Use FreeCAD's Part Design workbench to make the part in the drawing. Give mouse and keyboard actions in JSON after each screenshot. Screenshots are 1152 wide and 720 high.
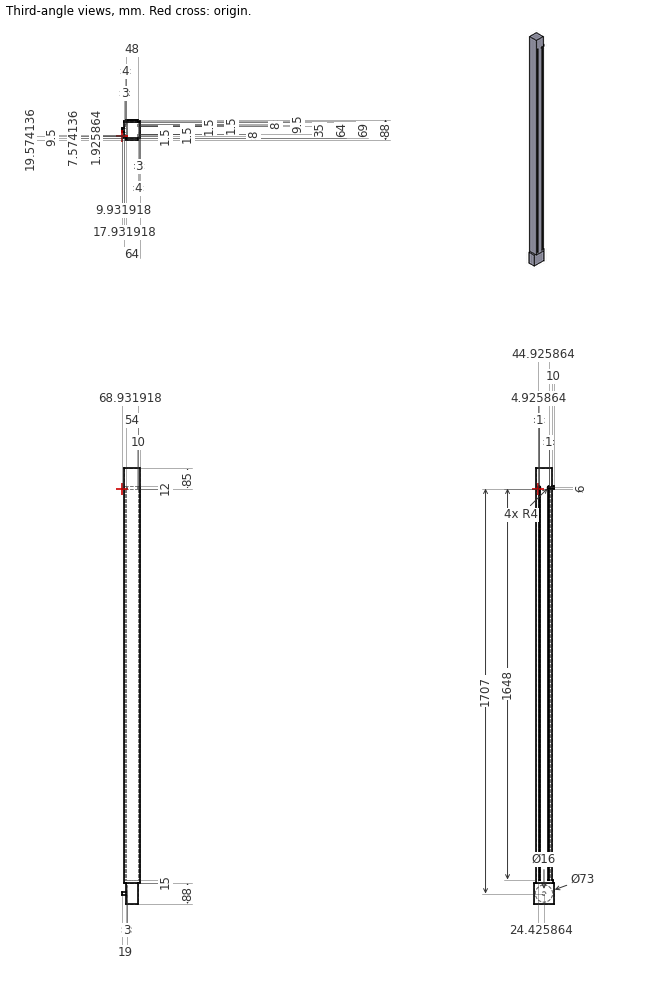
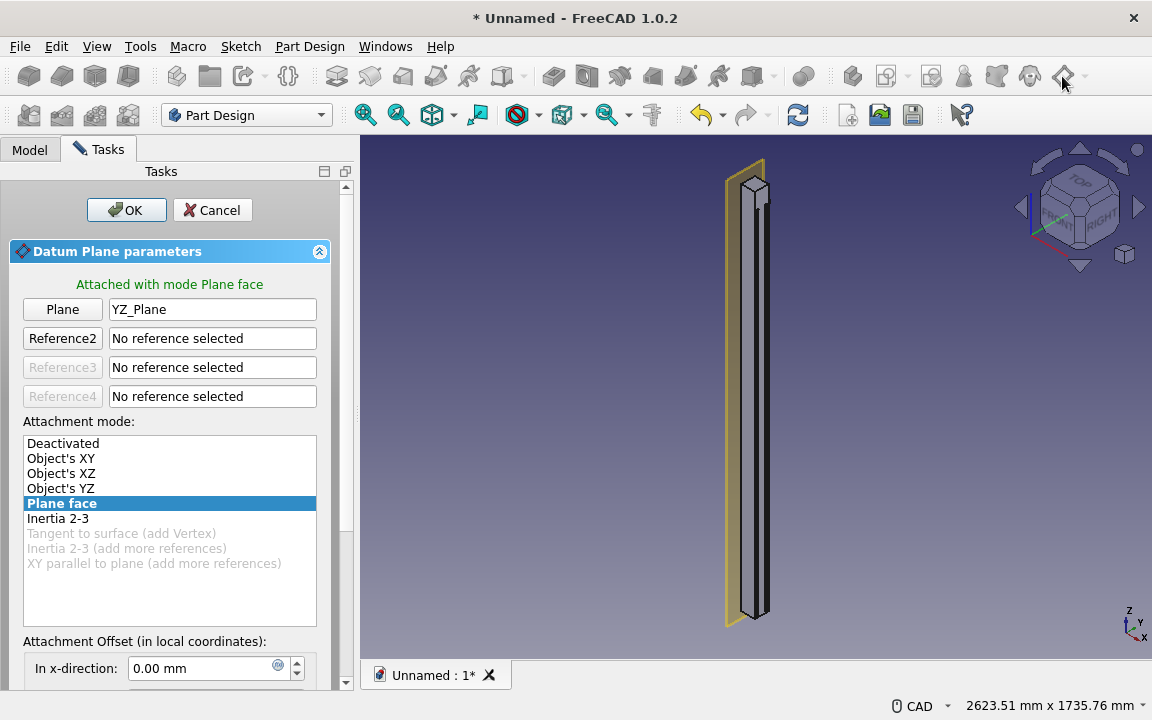
{"action": "scroll", "coordinate": [346, 436], "scroll_direction": "down", "scroll_amount": 2}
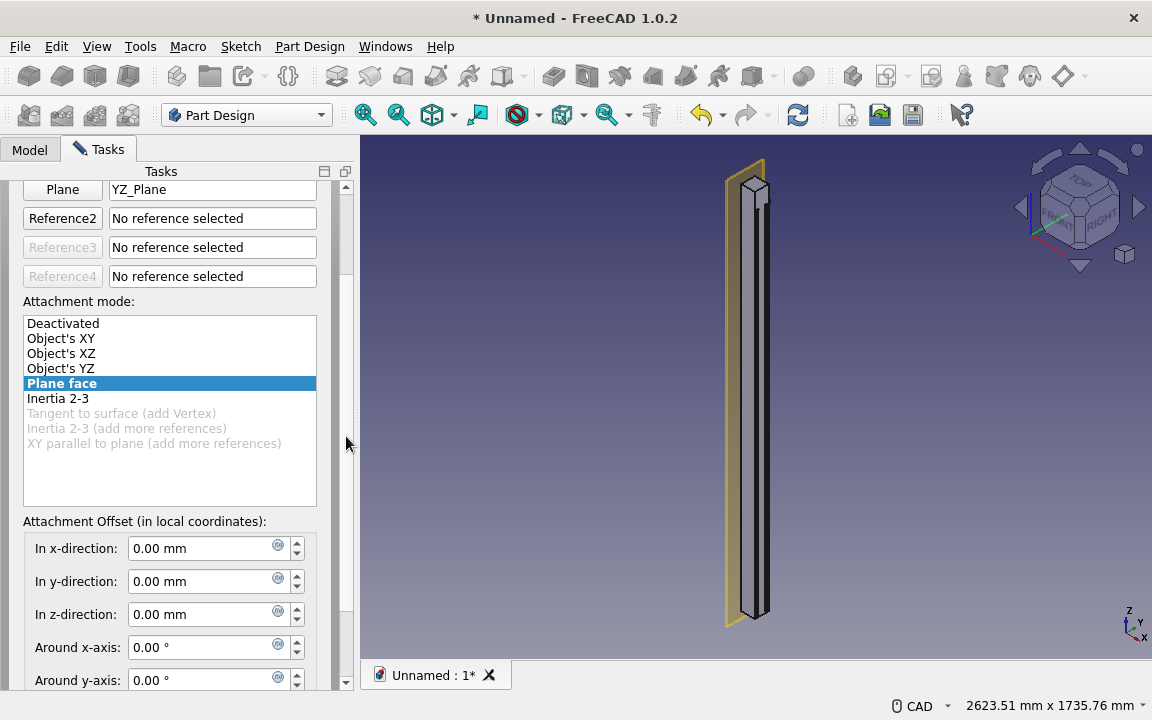
{"action": "triple_click", "coordinate": [210, 614]}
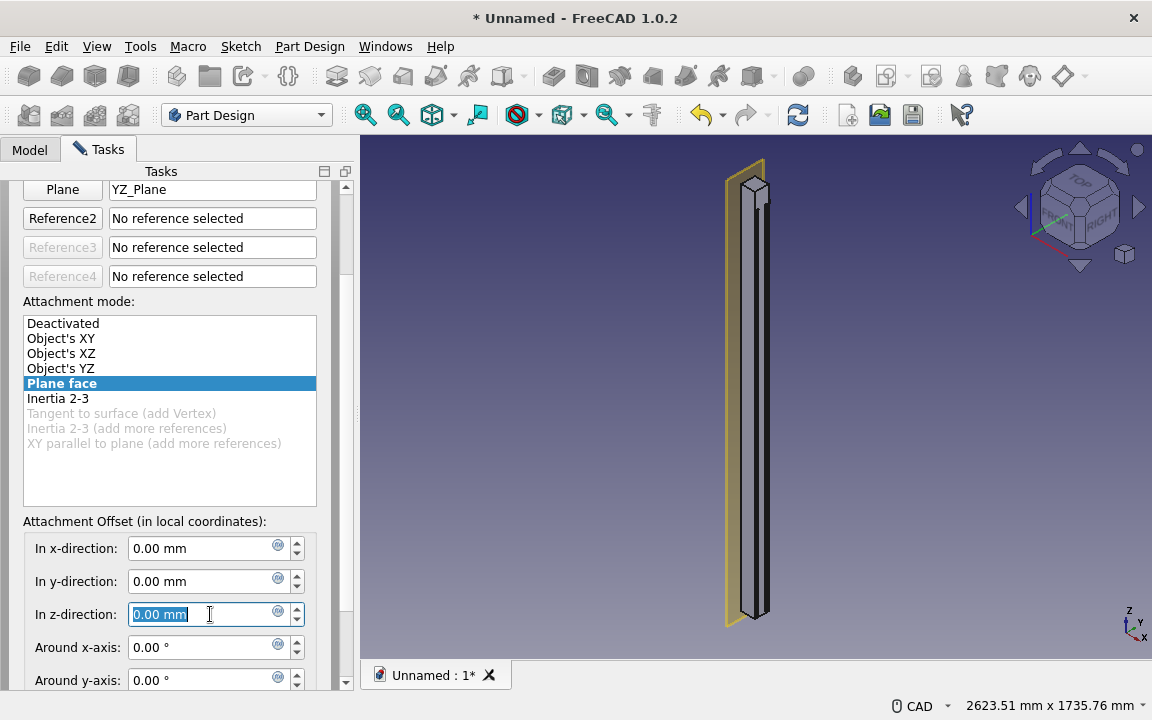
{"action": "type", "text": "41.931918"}
{"action": "key", "text": "Tab"}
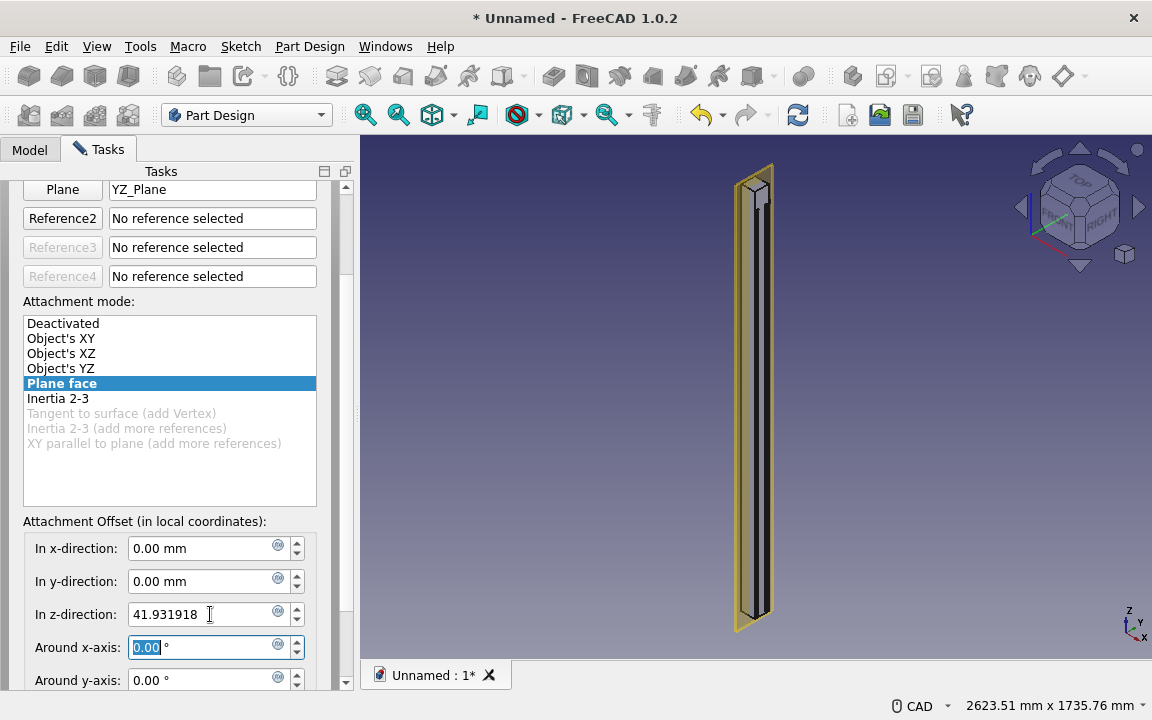
{"action": "scroll", "coordinate": [346, 436], "scroll_direction": "up", "scroll_amount": 3}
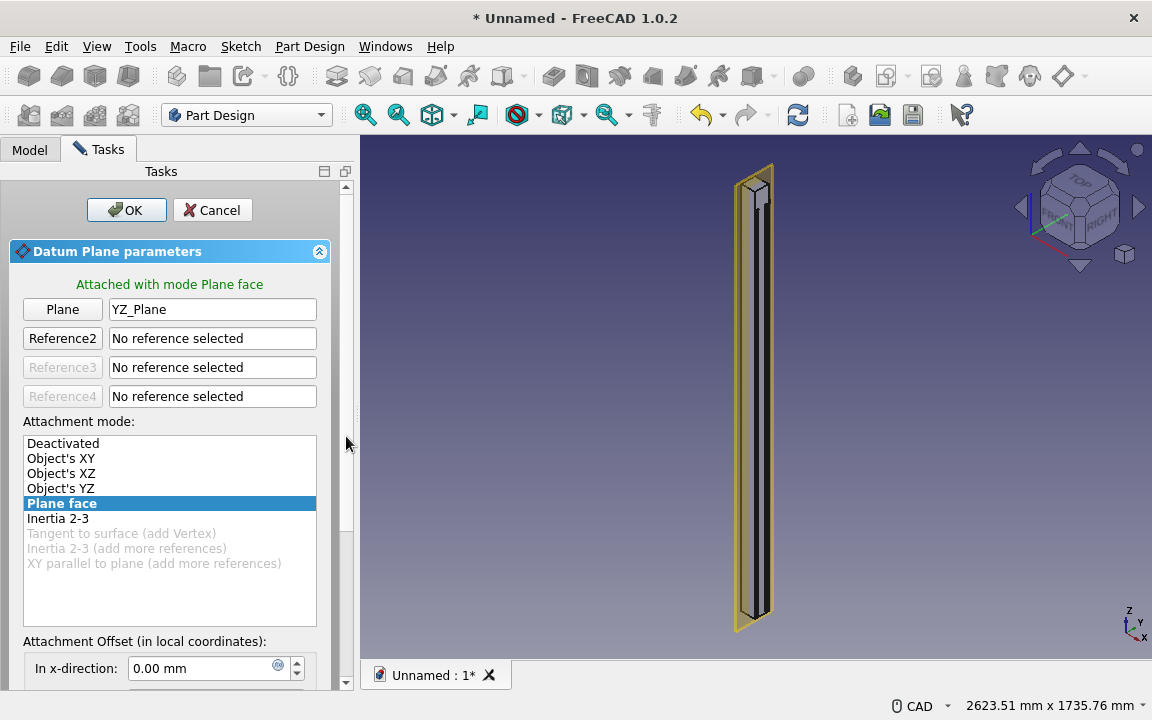
{"action": "left_click", "coordinate": [127, 210]}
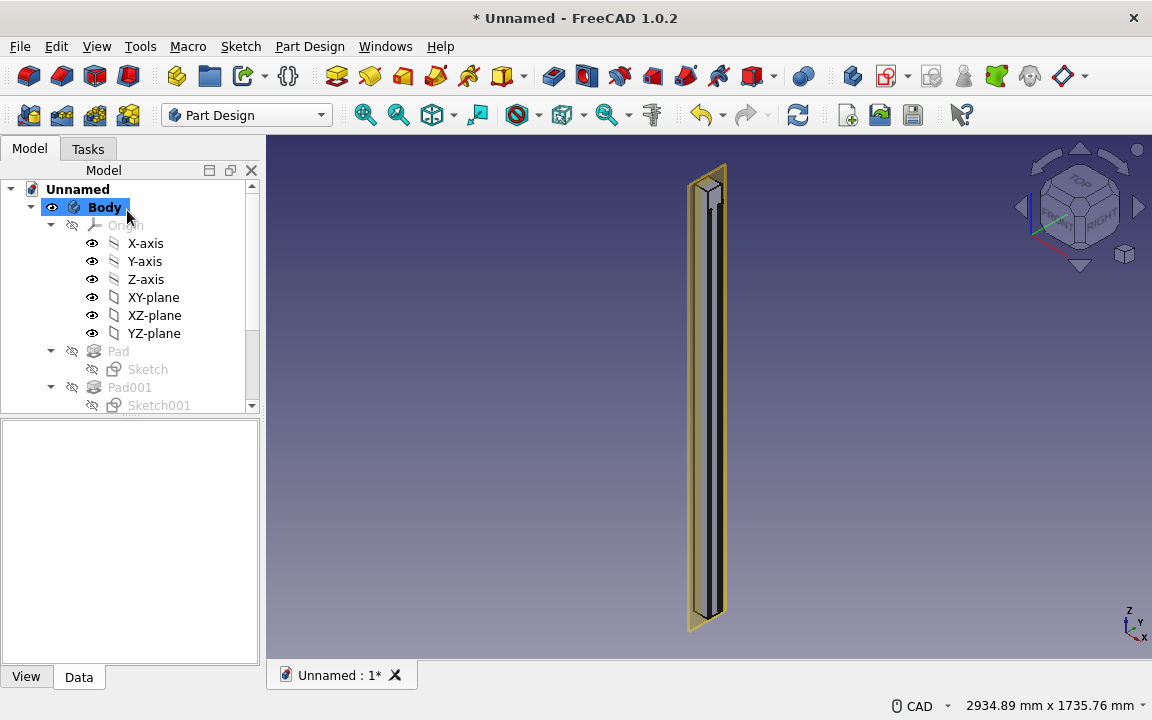
{"action": "scroll", "coordinate": [101, 293], "scroll_direction": "down", "scroll_amount": 3}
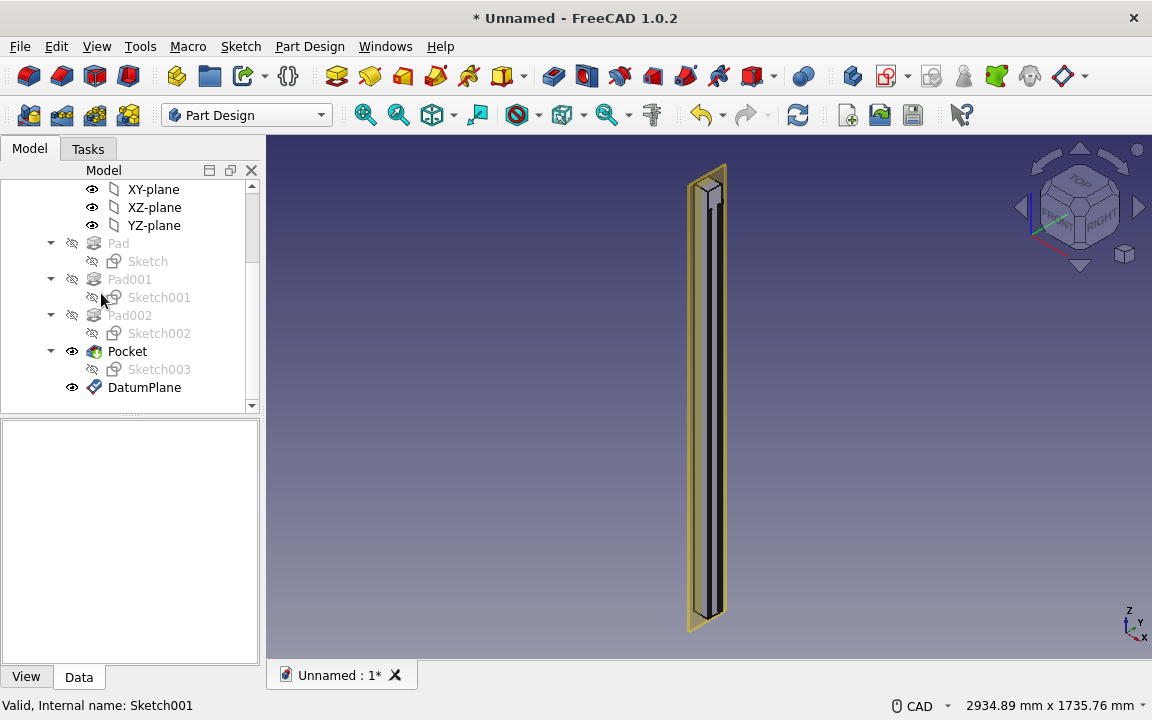
{"action": "left_click", "coordinate": [117, 351]}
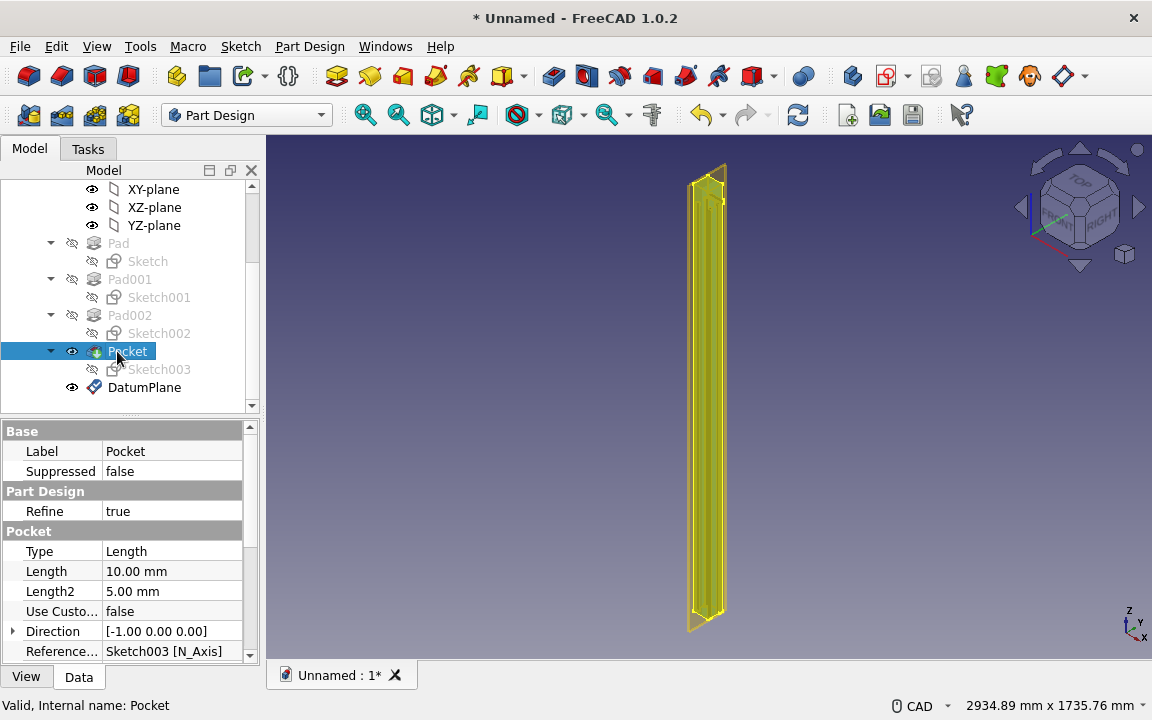
{"action": "left_click", "coordinate": [29, 116]}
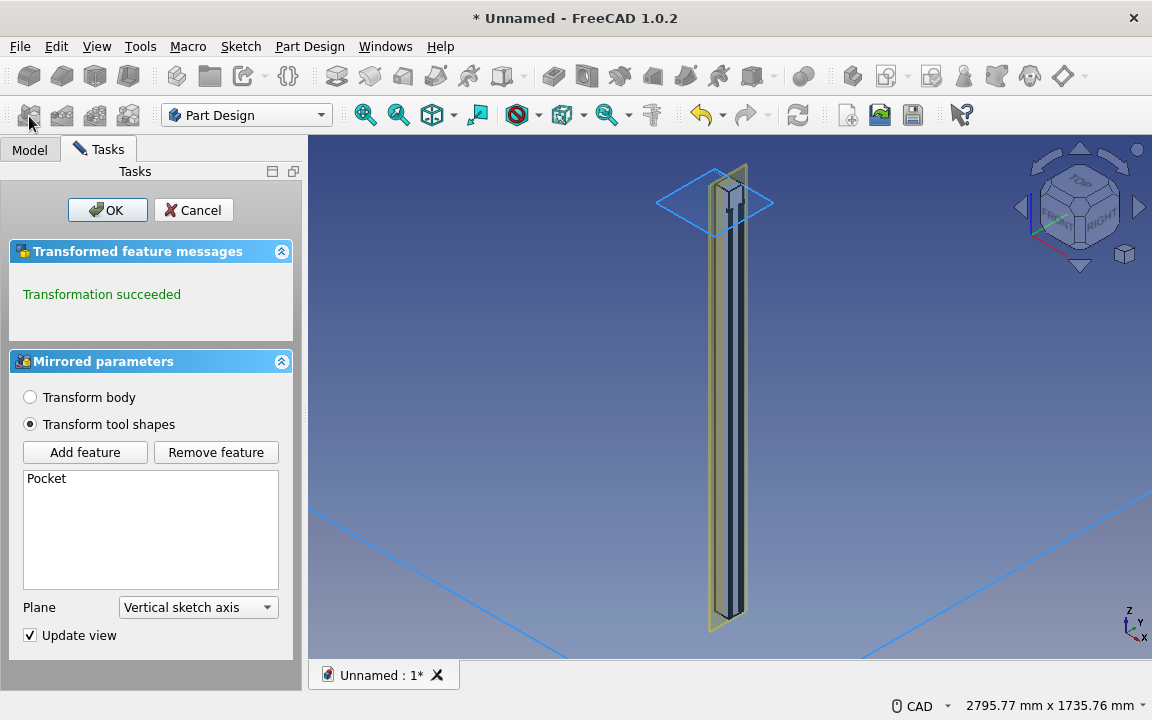
{"action": "left_click", "coordinate": [199, 608]}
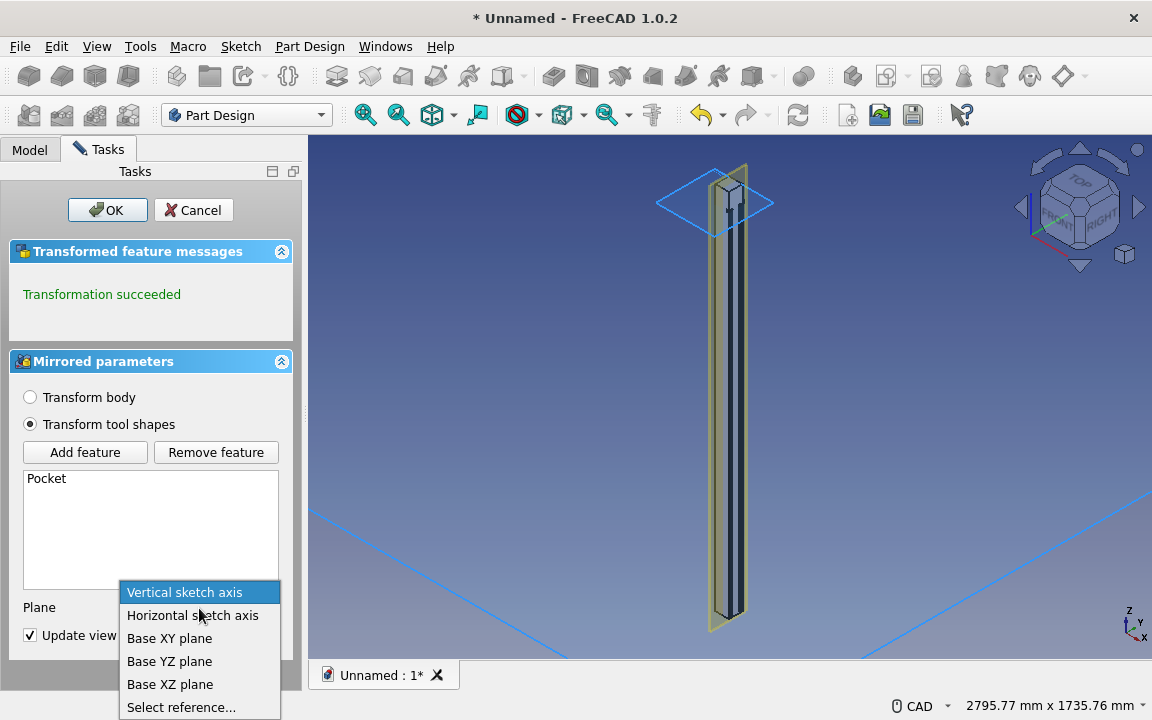
{"action": "left_click", "coordinate": [198, 708]}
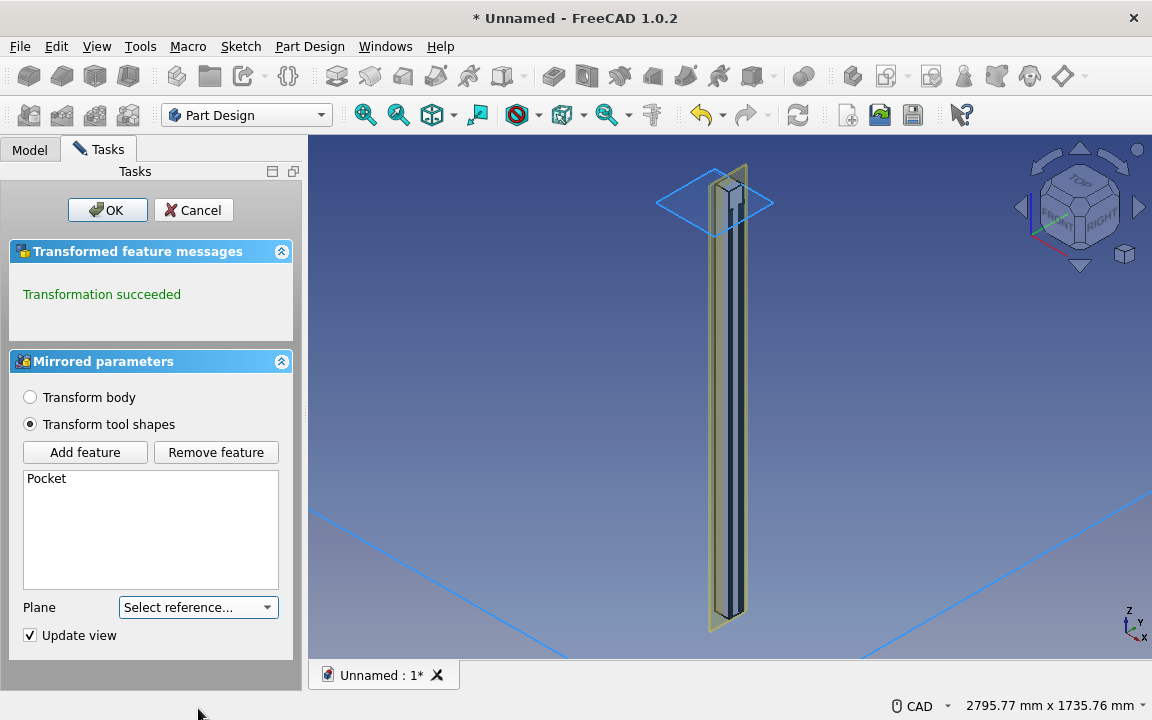
{"action": "left_click", "coordinate": [30, 149]}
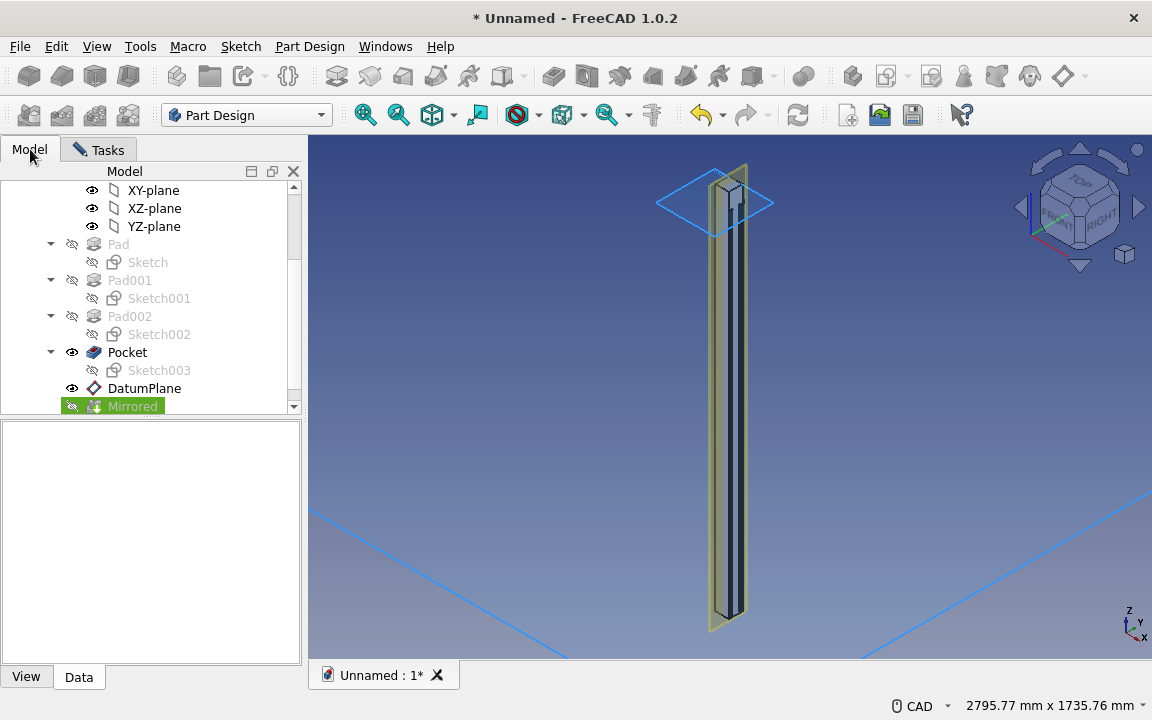
{"action": "left_click", "coordinate": [117, 388]}